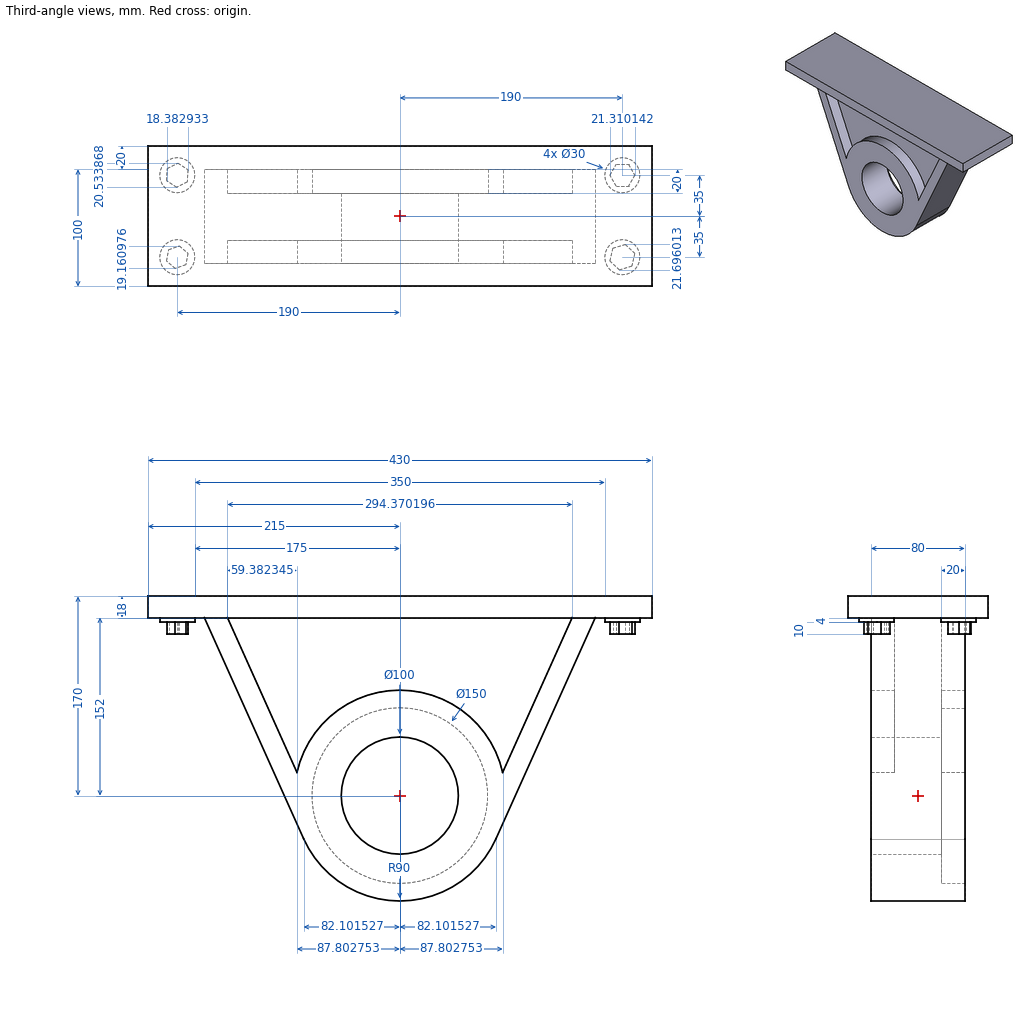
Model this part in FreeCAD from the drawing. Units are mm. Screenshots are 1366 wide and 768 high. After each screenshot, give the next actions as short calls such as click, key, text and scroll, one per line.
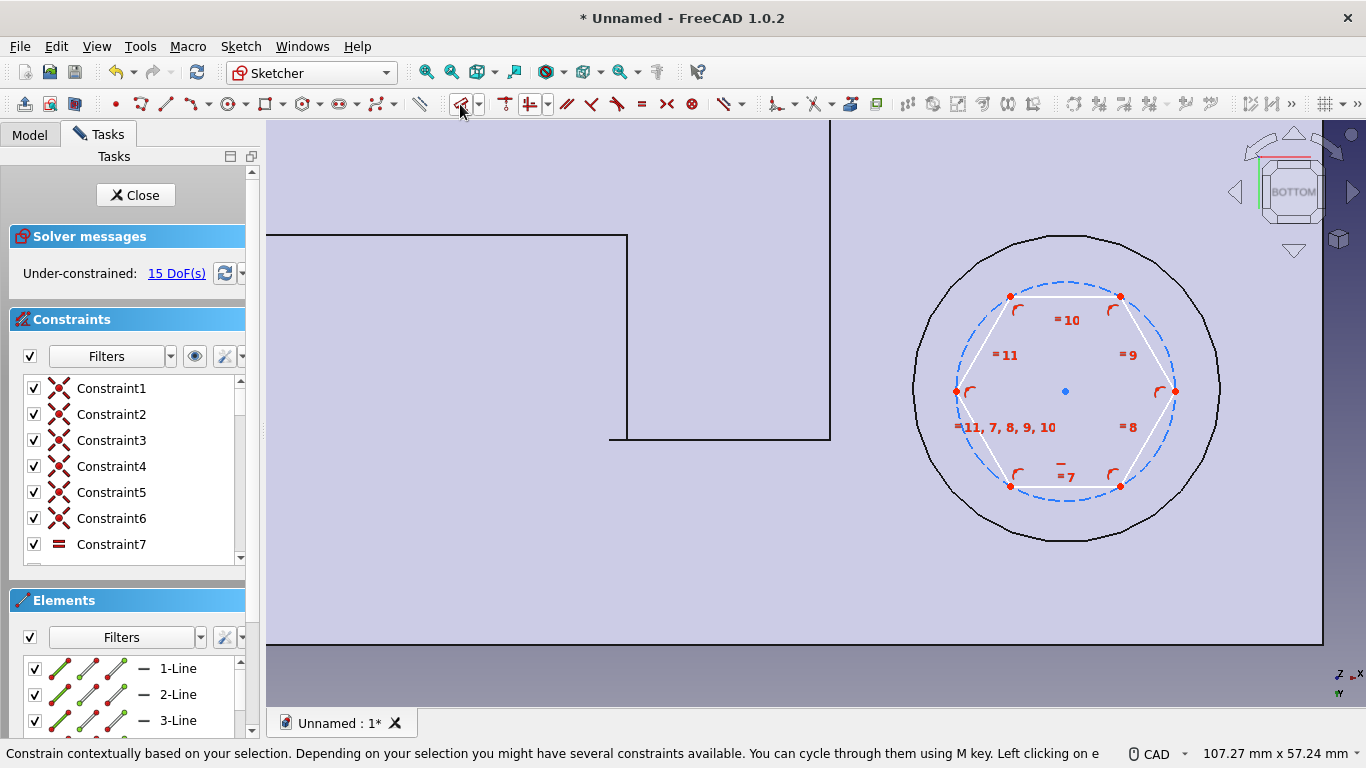
scroll(1069, 490, down, 9)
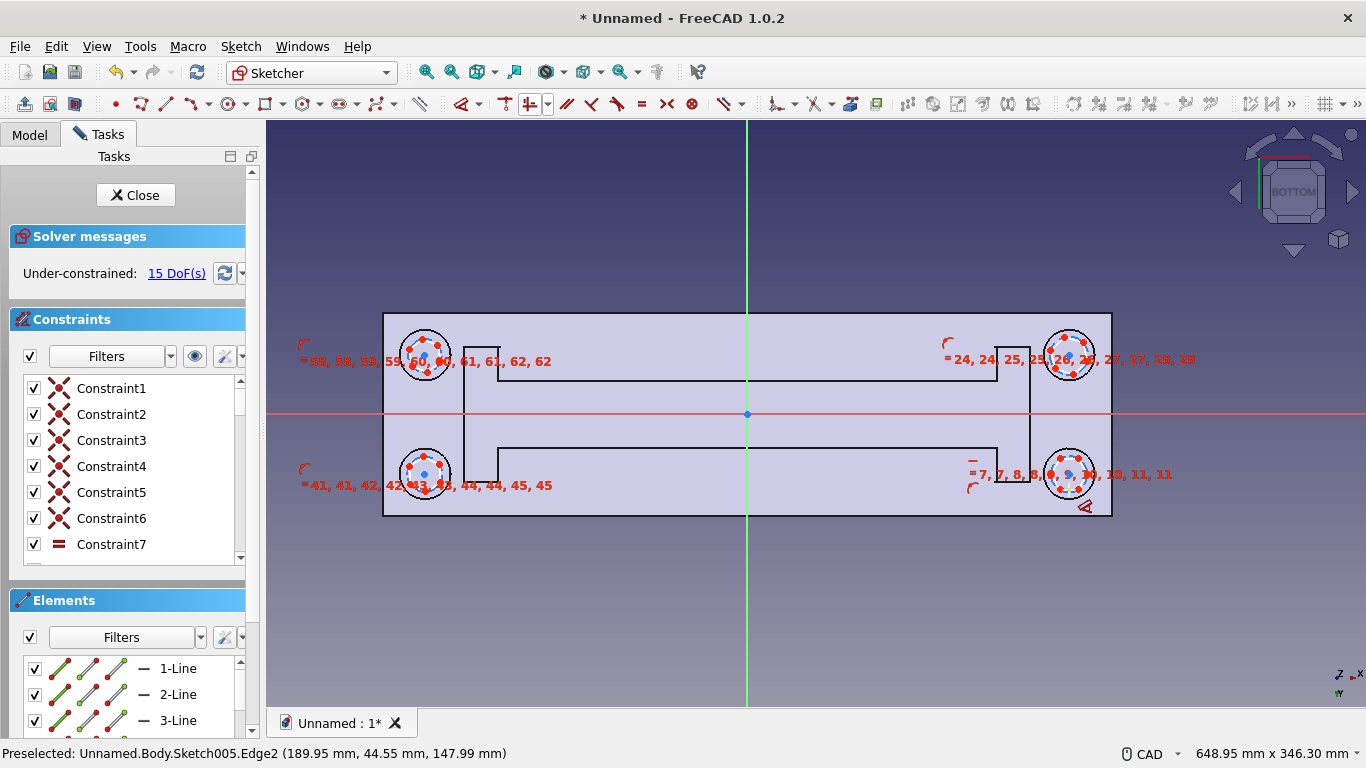
click(1069, 474)
click(1103, 444)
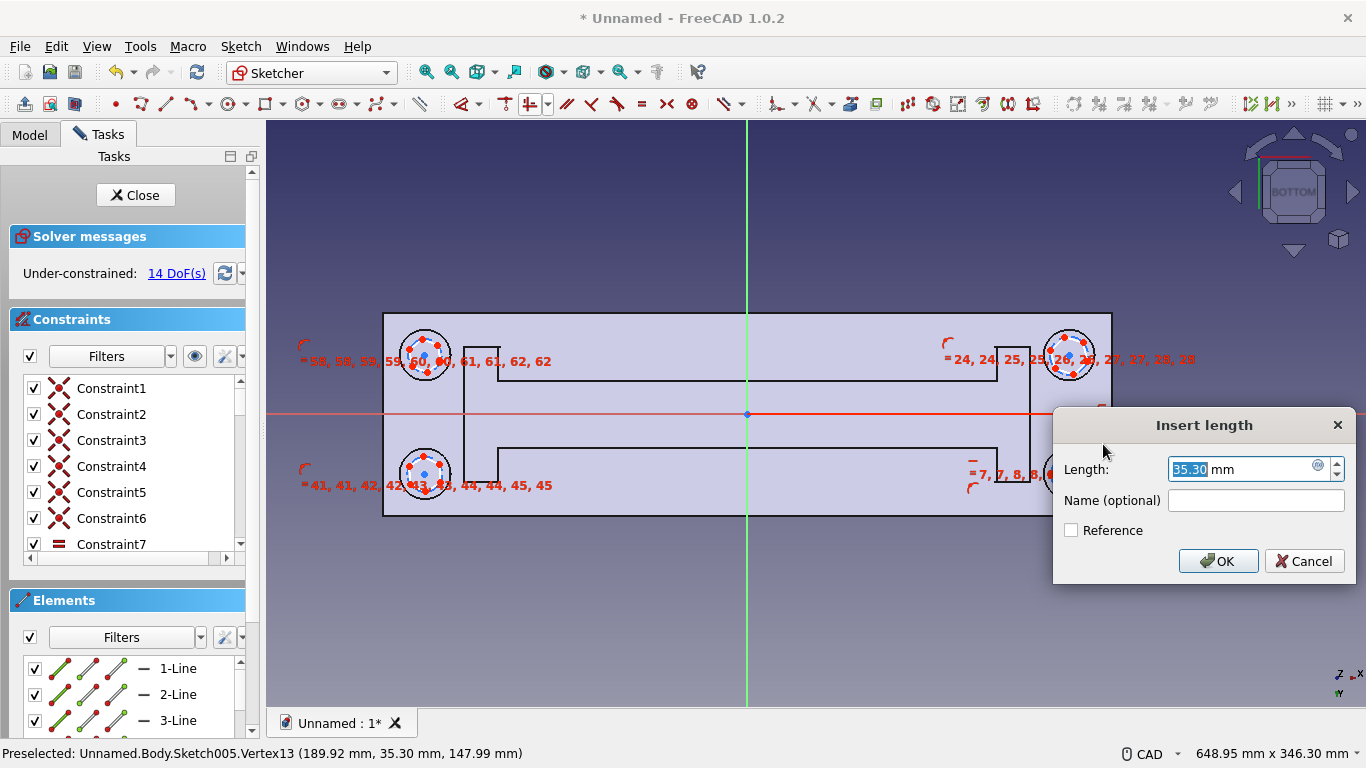
text(35)
key(Return)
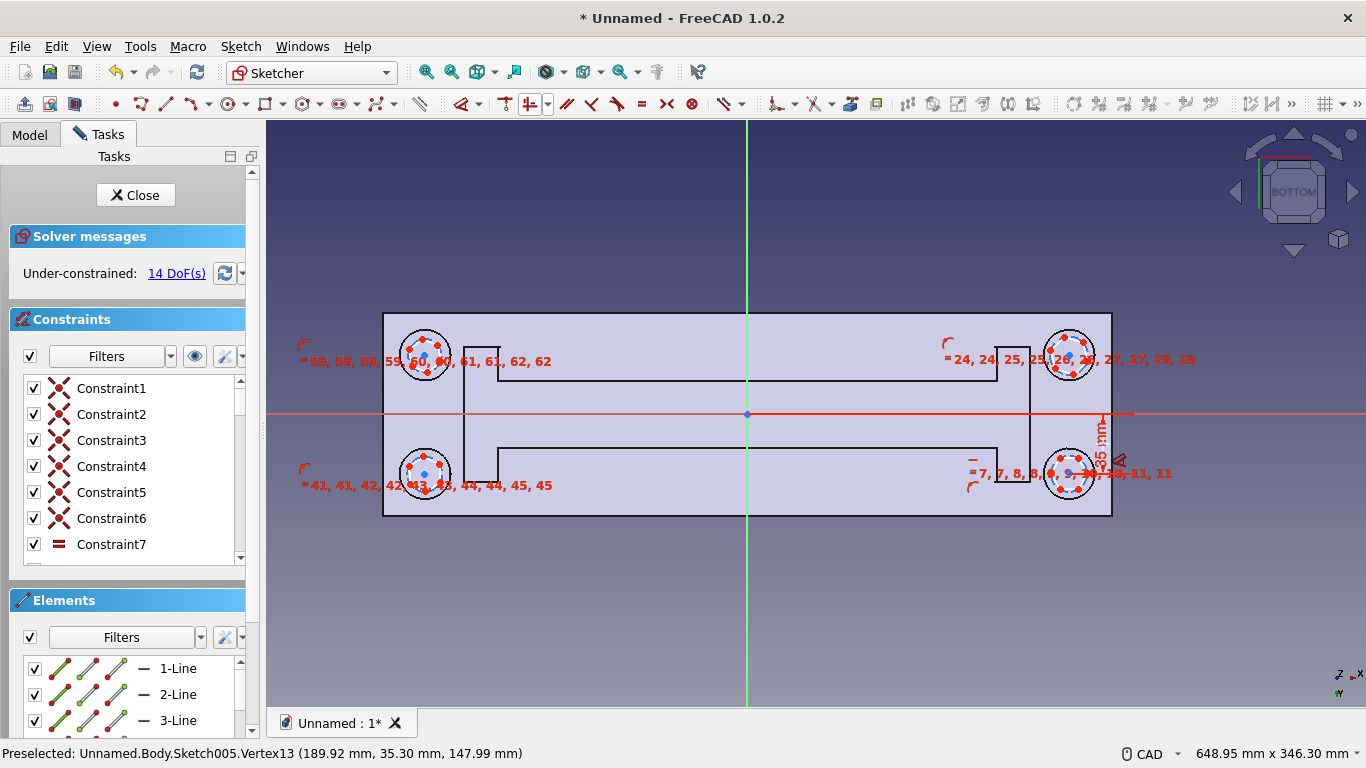
click(1069, 356)
click(1103, 385)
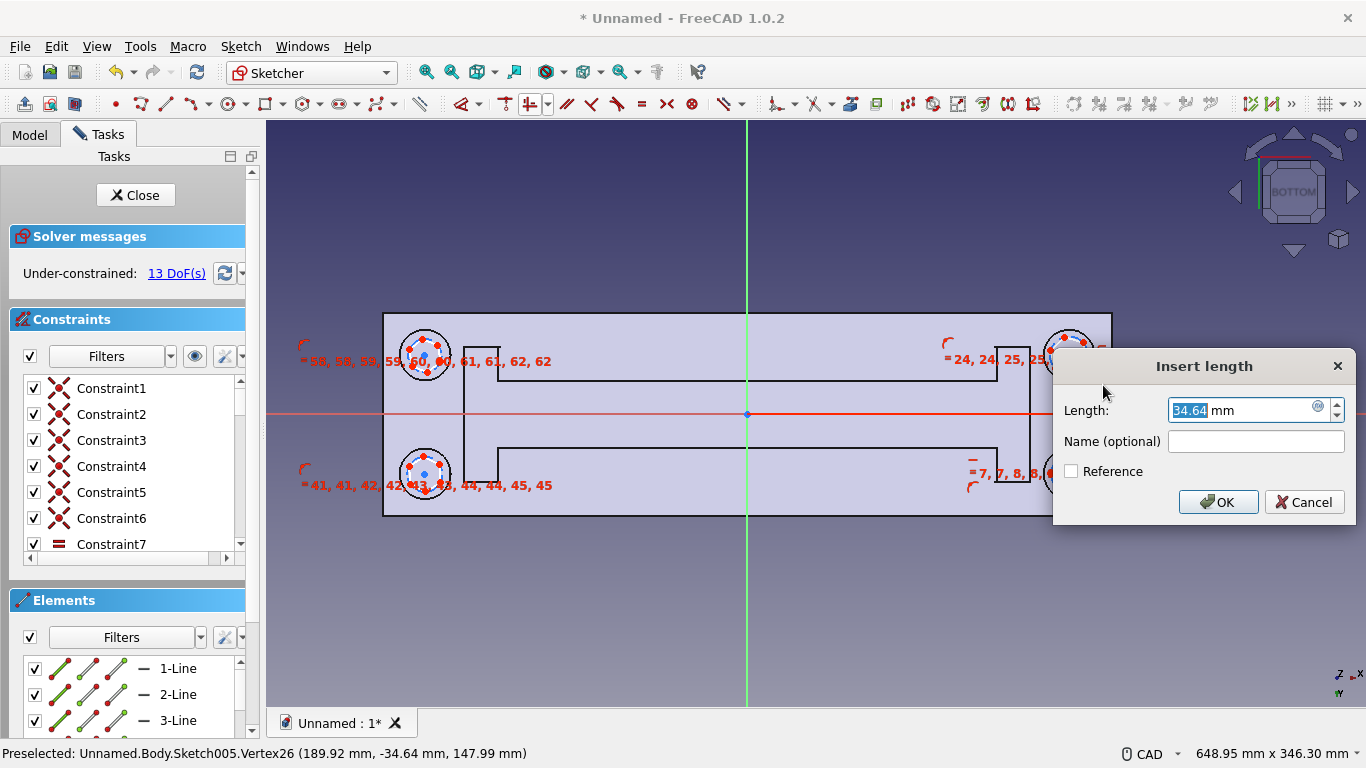
text(35)
key(Return)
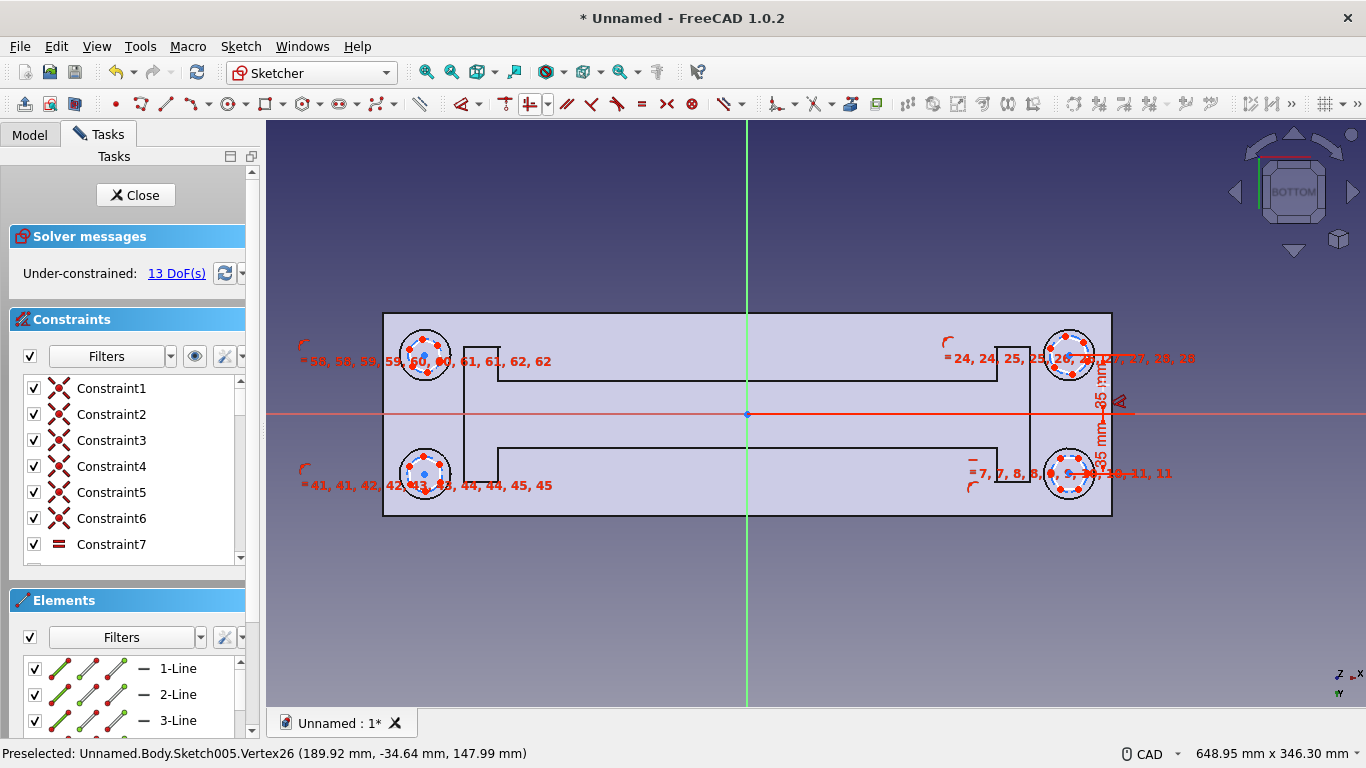
click(425, 474)
click(391, 444)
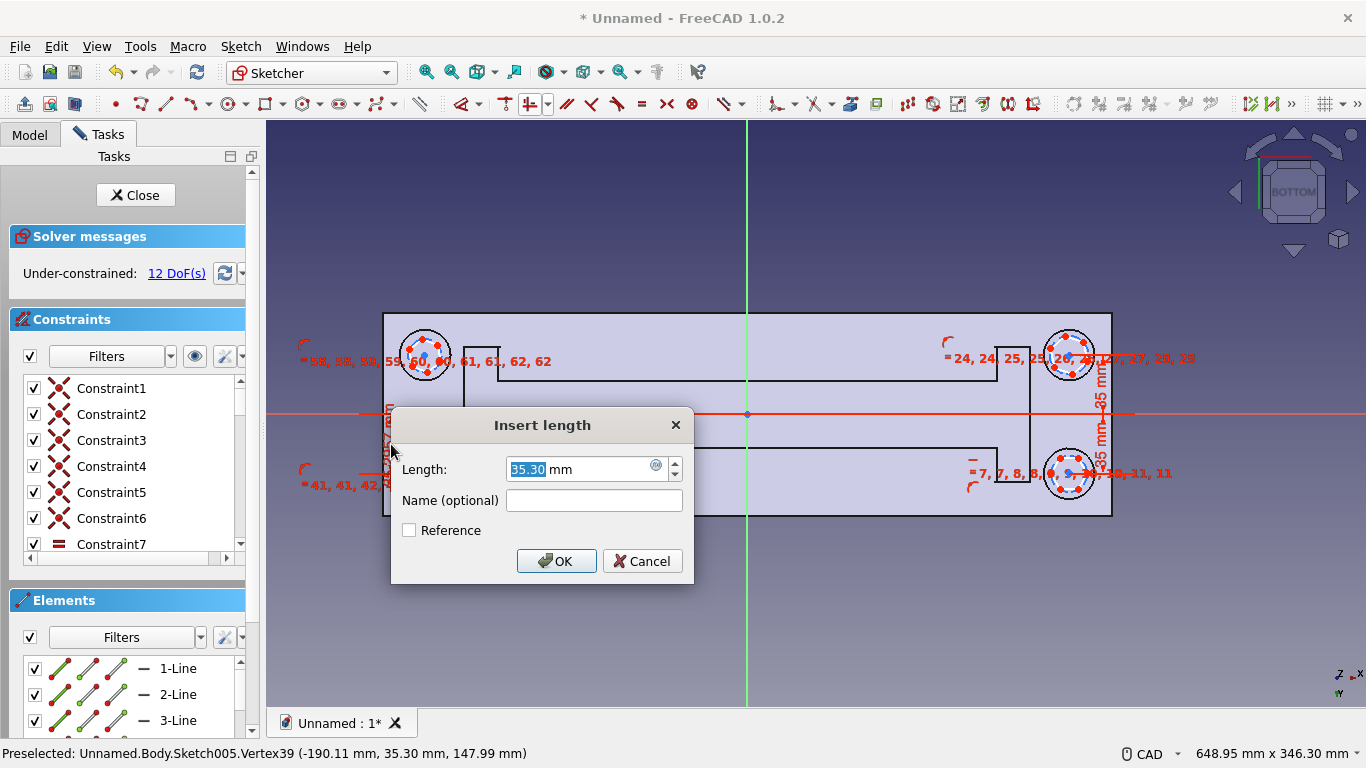
text(35)
key(Return)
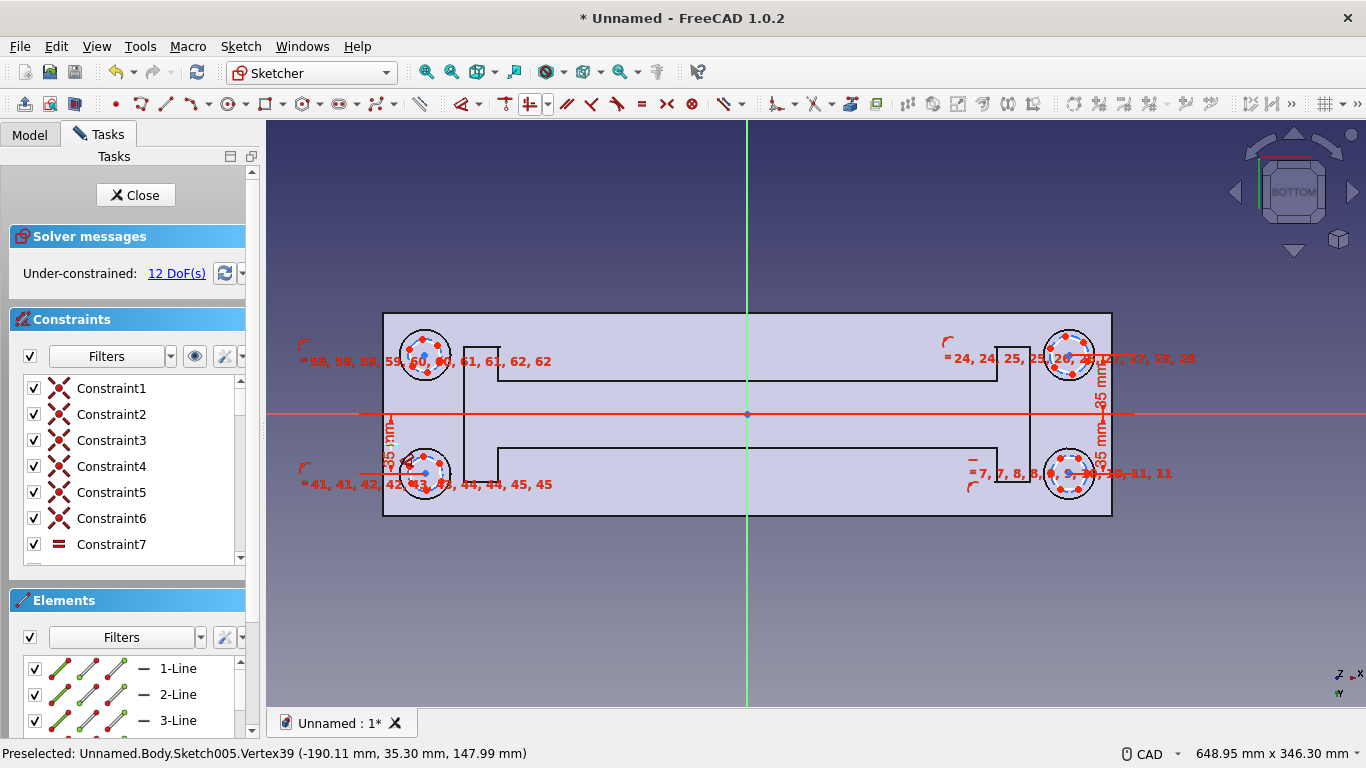
click(425, 356)
click(391, 385)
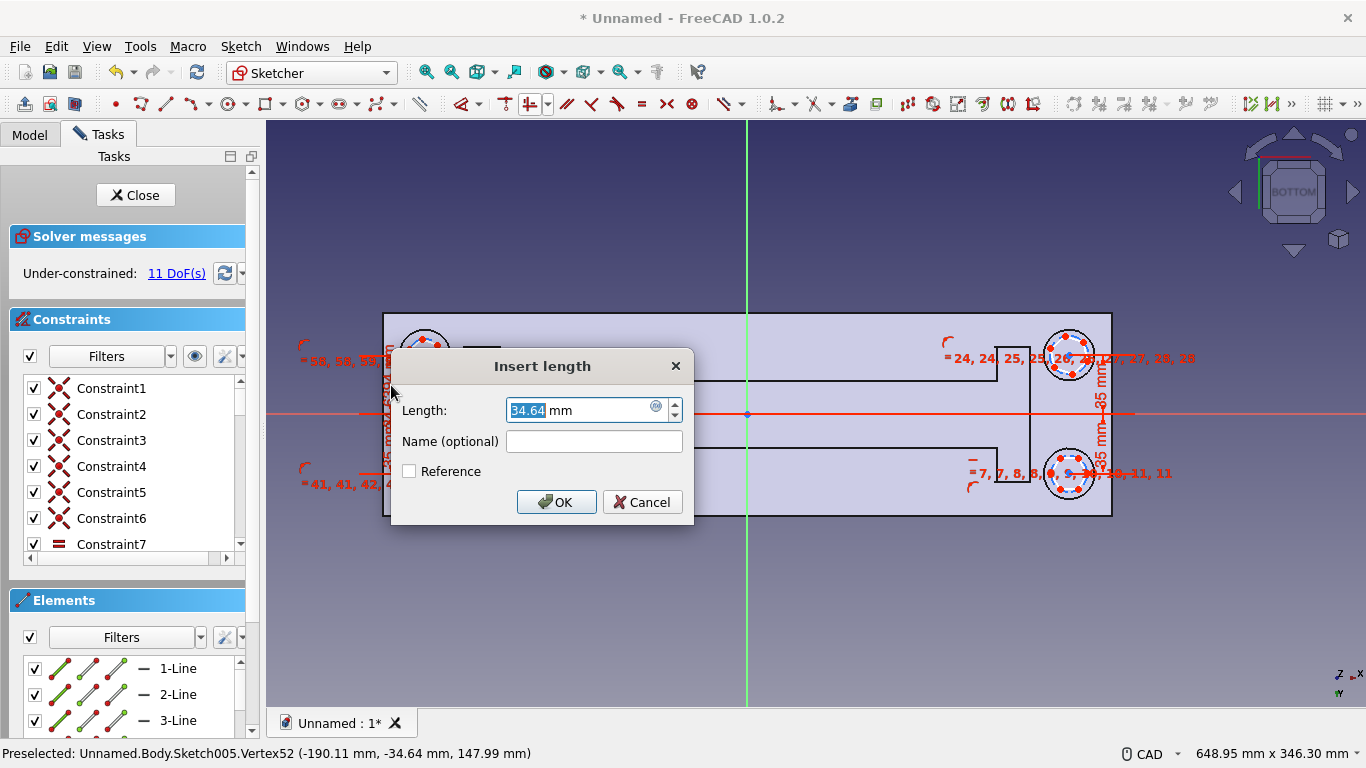
text(35)
key(Return)